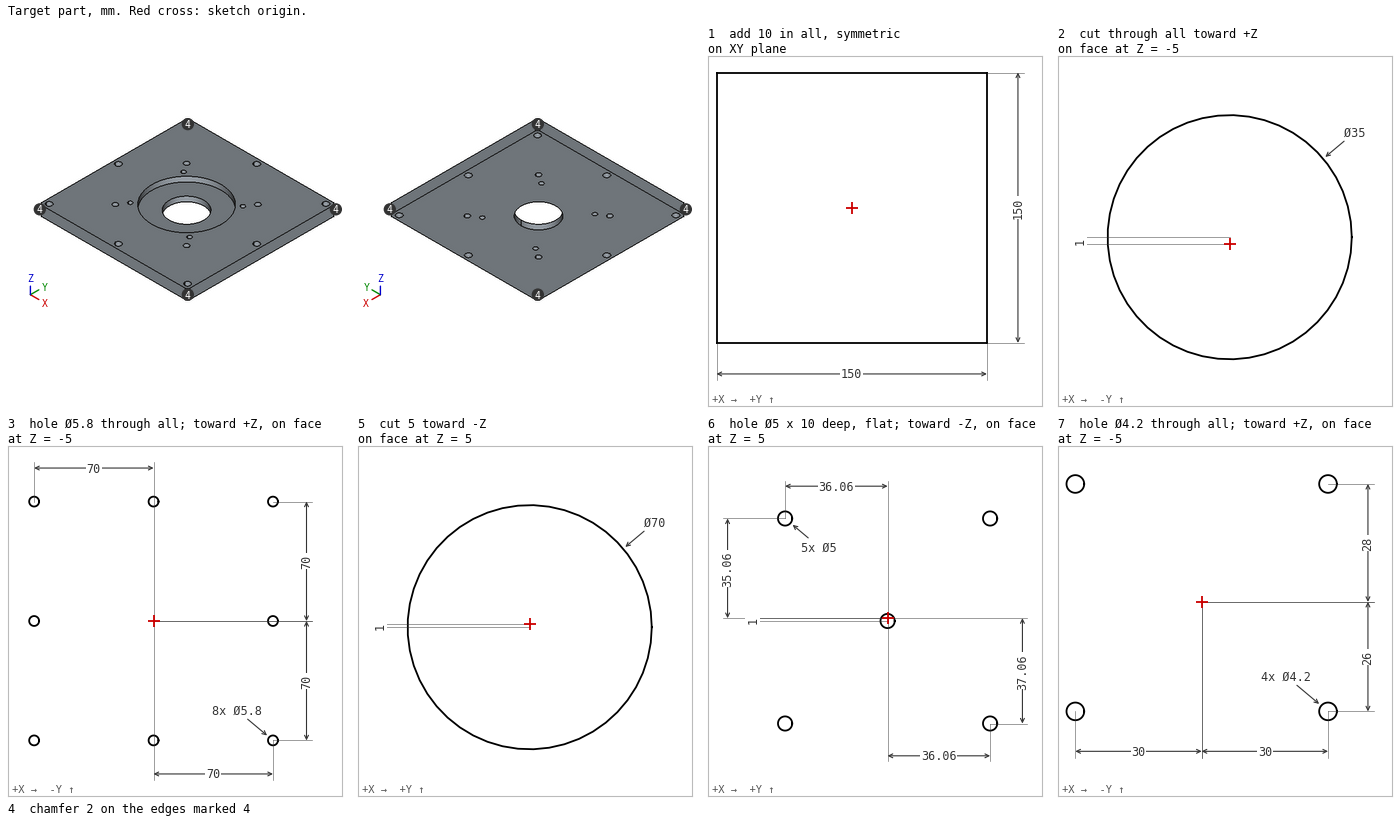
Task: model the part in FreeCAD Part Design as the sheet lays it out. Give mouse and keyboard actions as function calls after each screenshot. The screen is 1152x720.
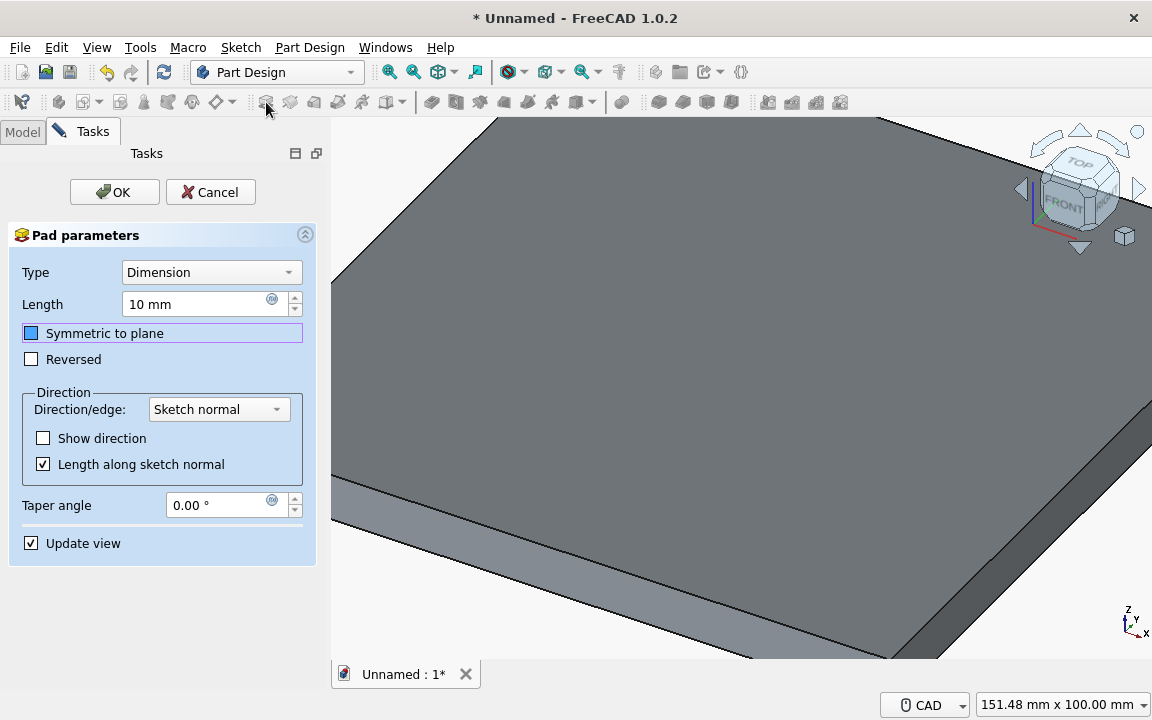
click(30, 333)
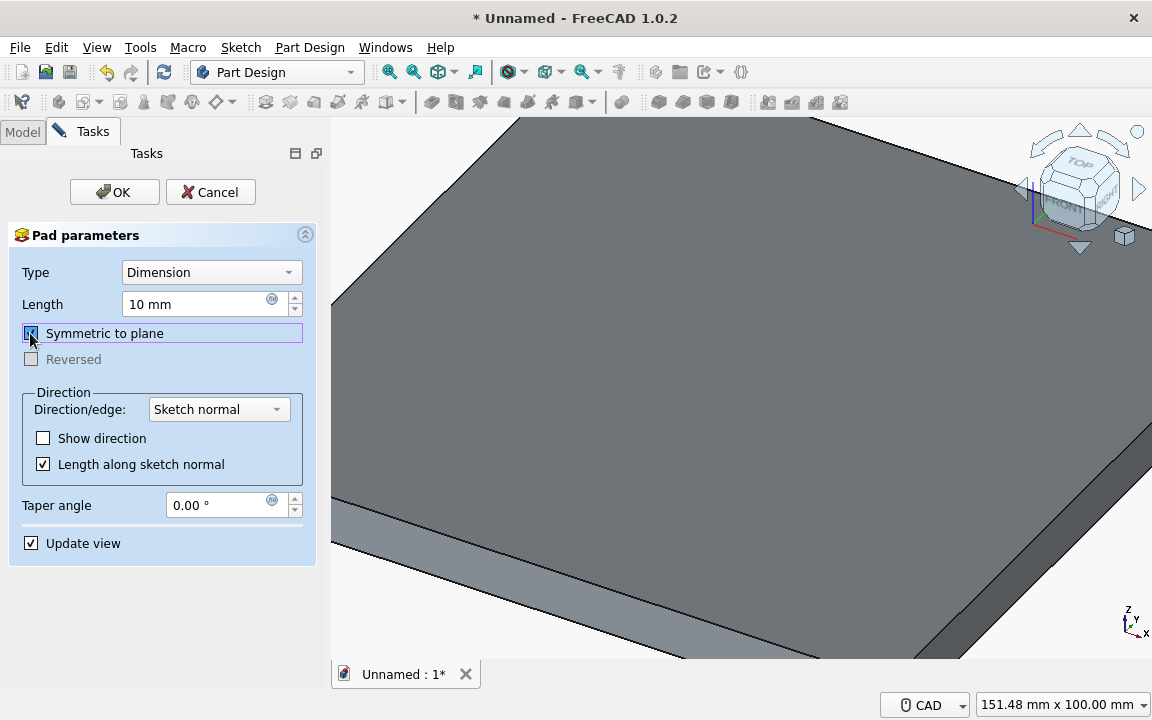
click(115, 192)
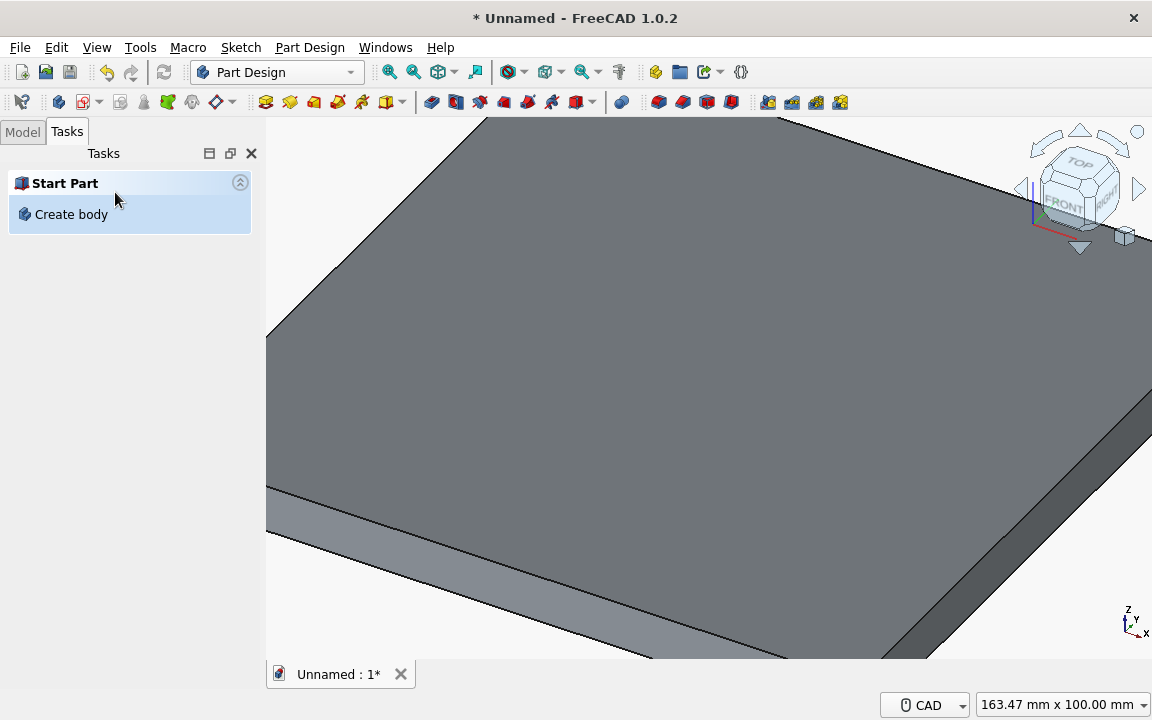
key(v)
key(f)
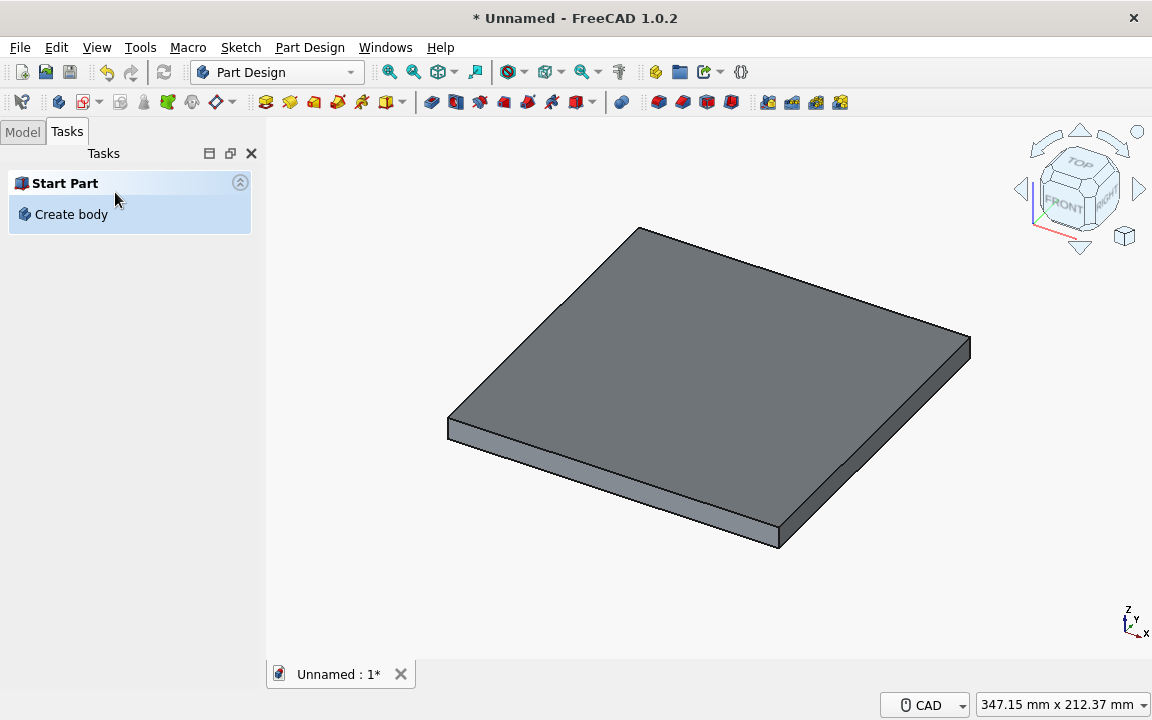
key(5)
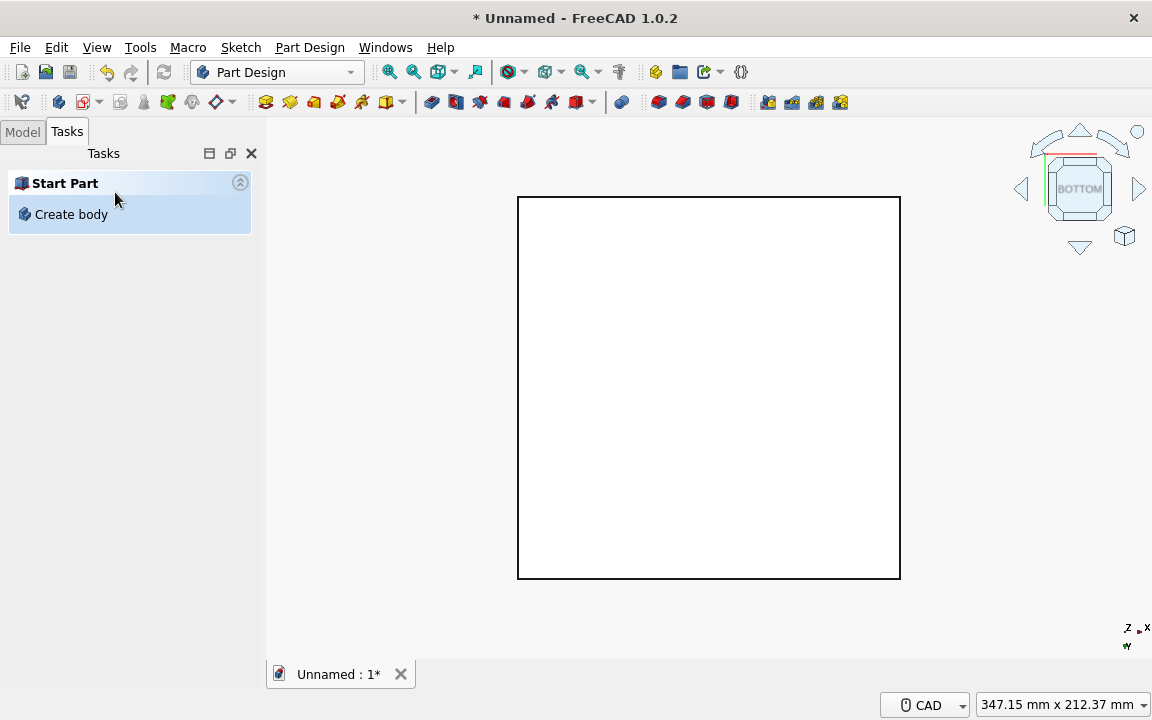
click(709, 387)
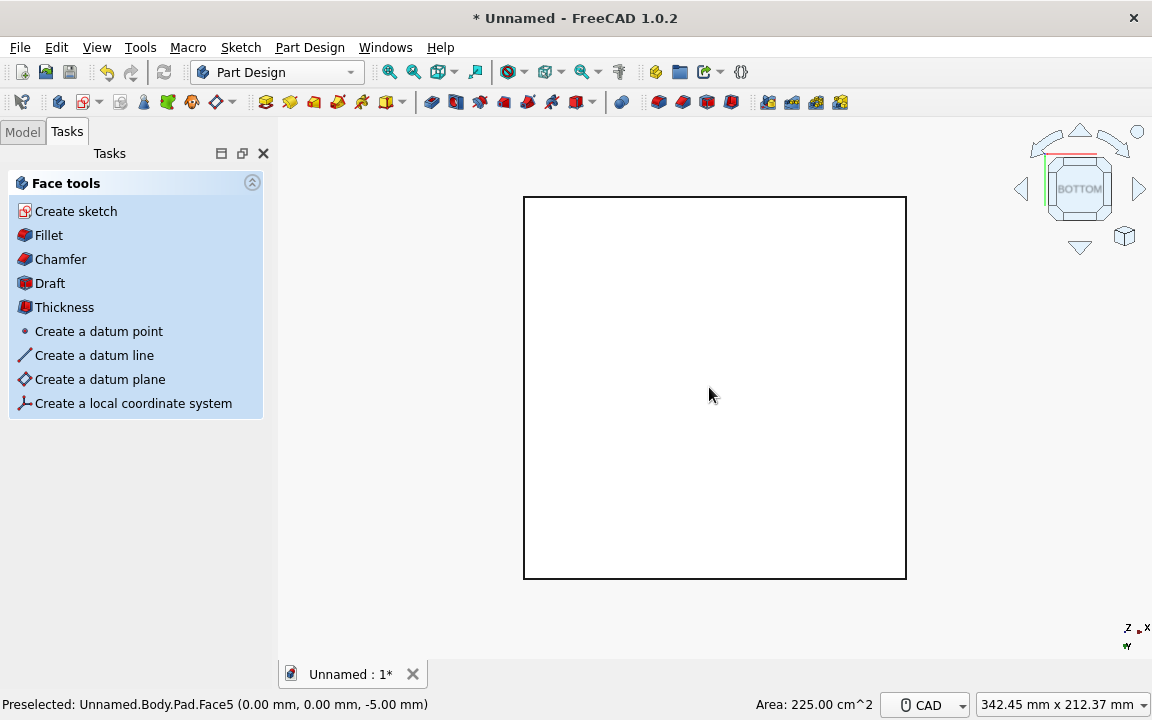
click(84, 102)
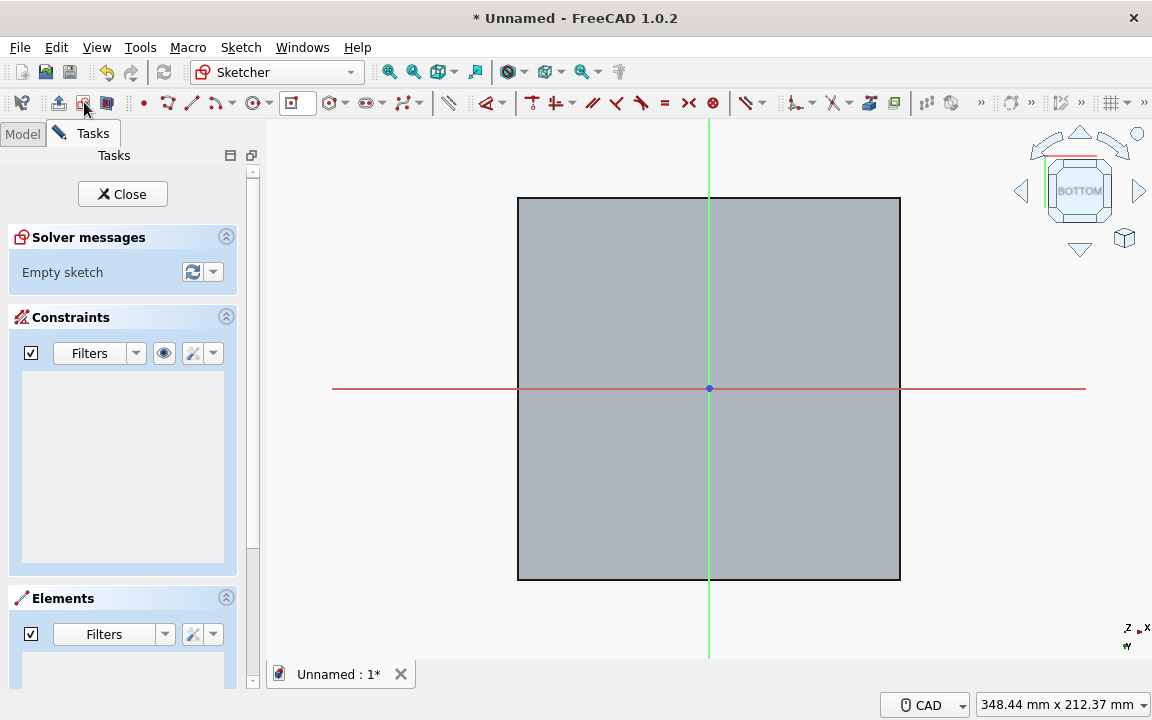
scroll(731, 386, up, 7)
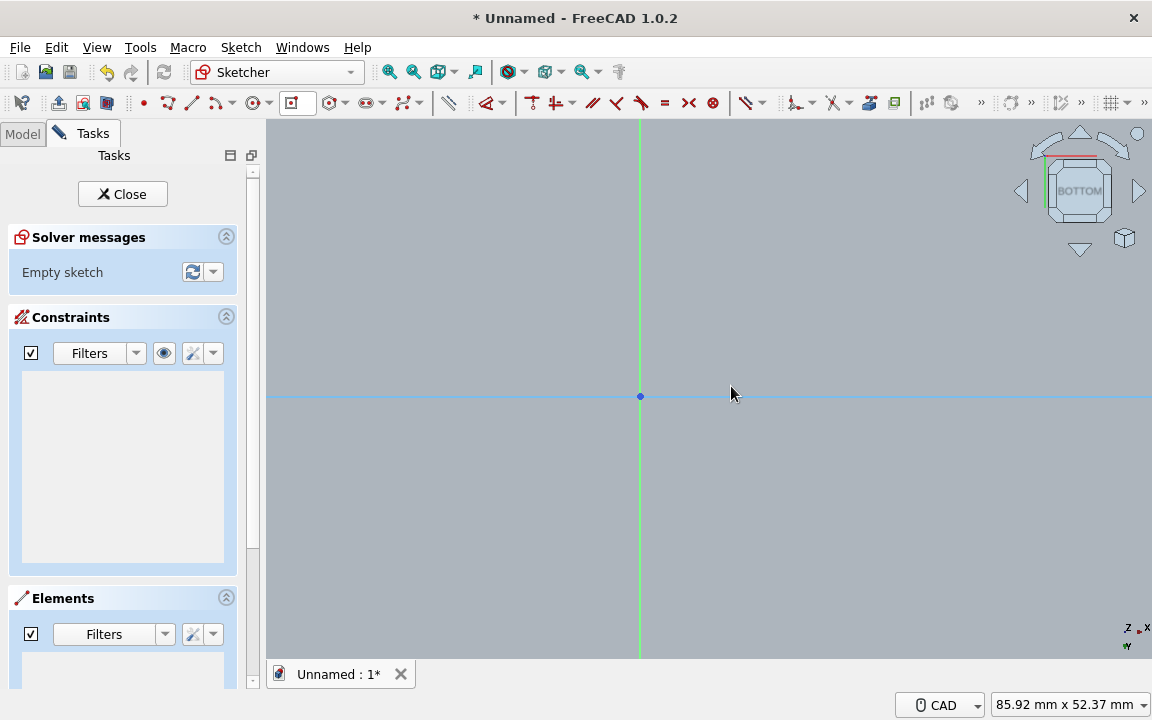
click(254, 104)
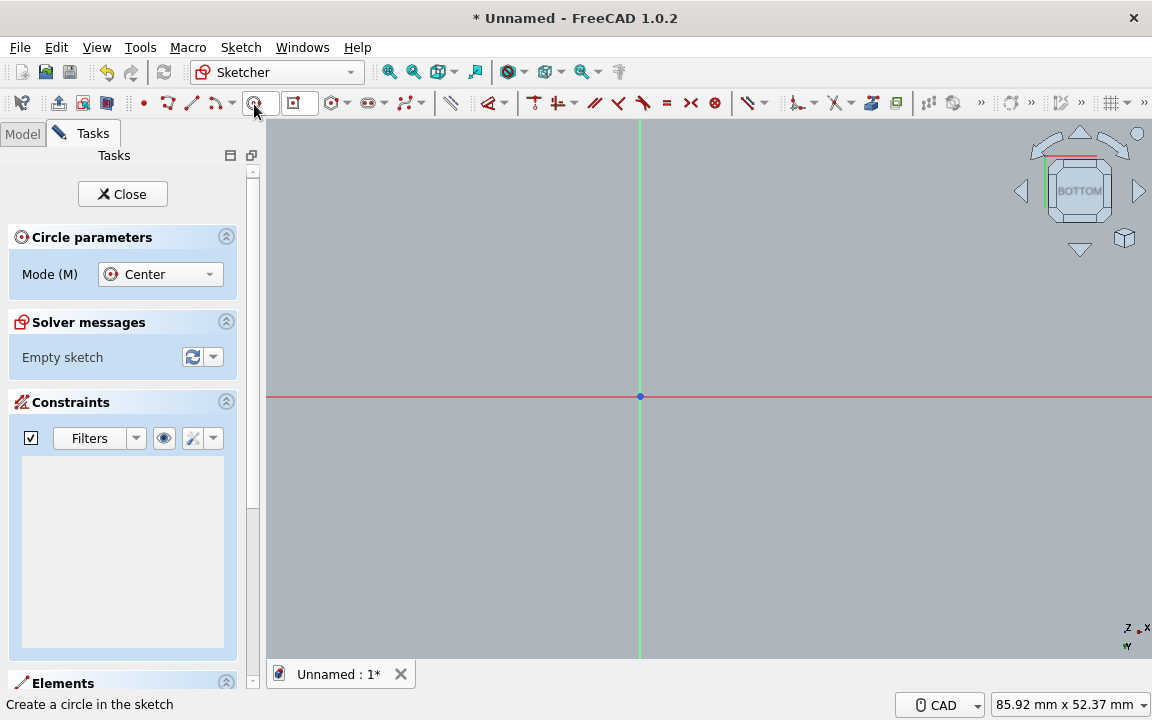
scroll(640, 386, up, 3)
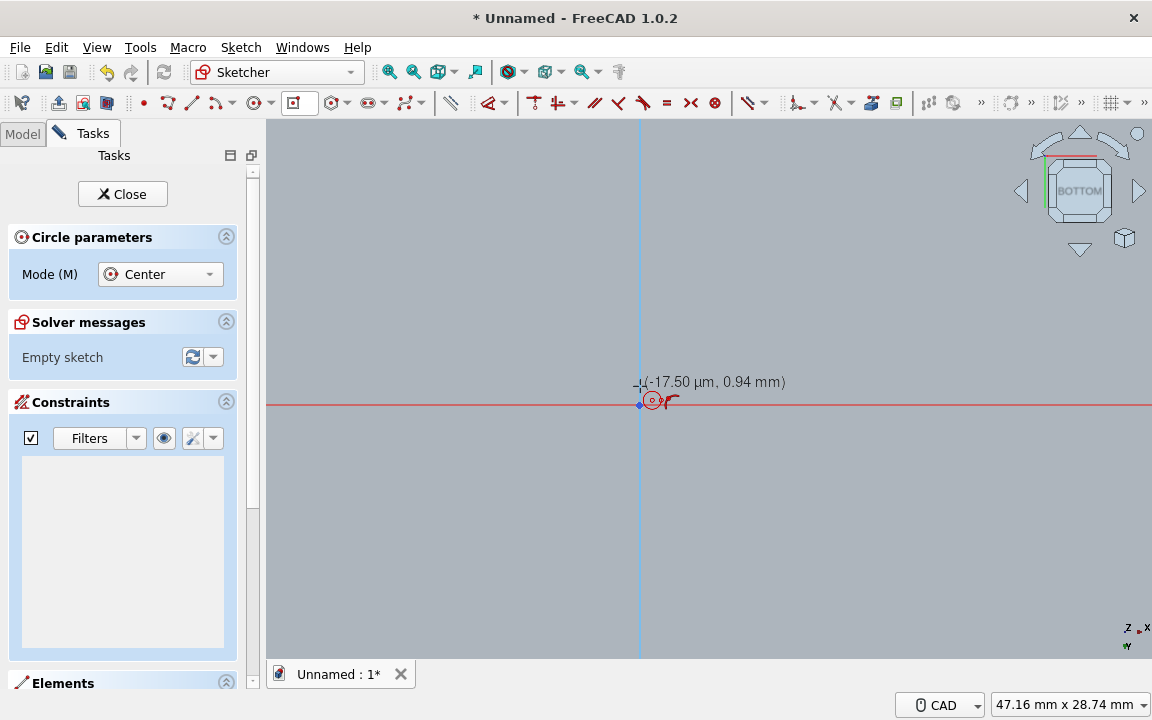
click(640, 386)
move(872, 154)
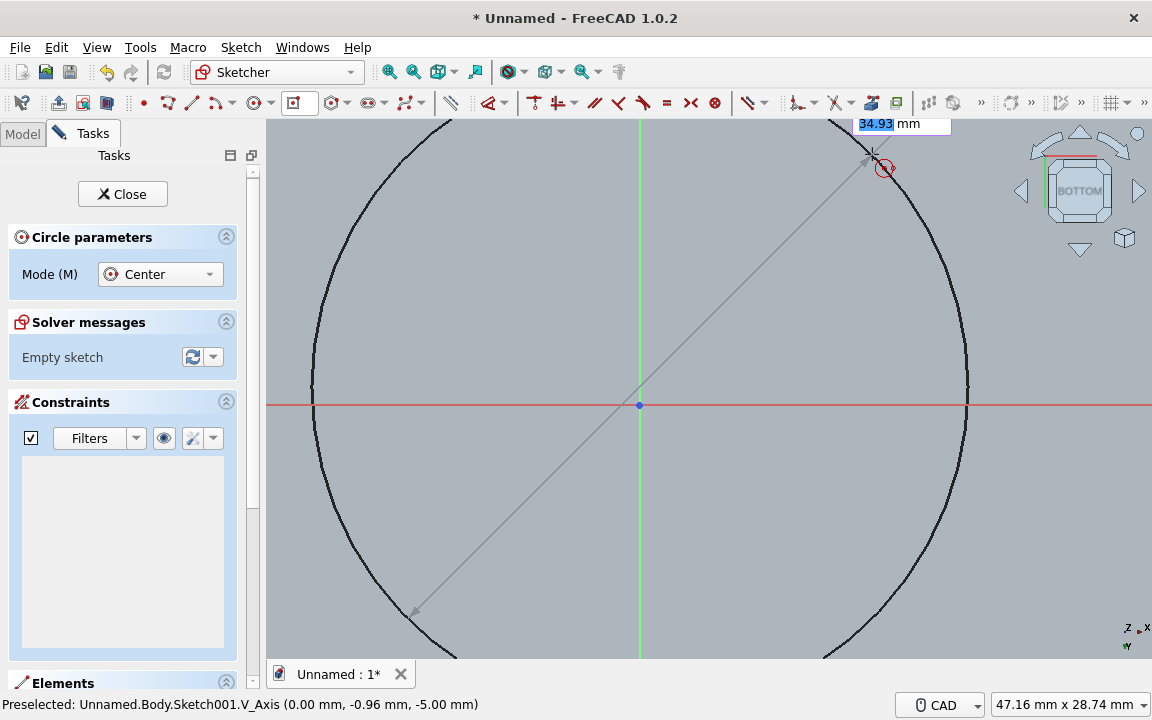
text(35)
key(Return)
key(Escape)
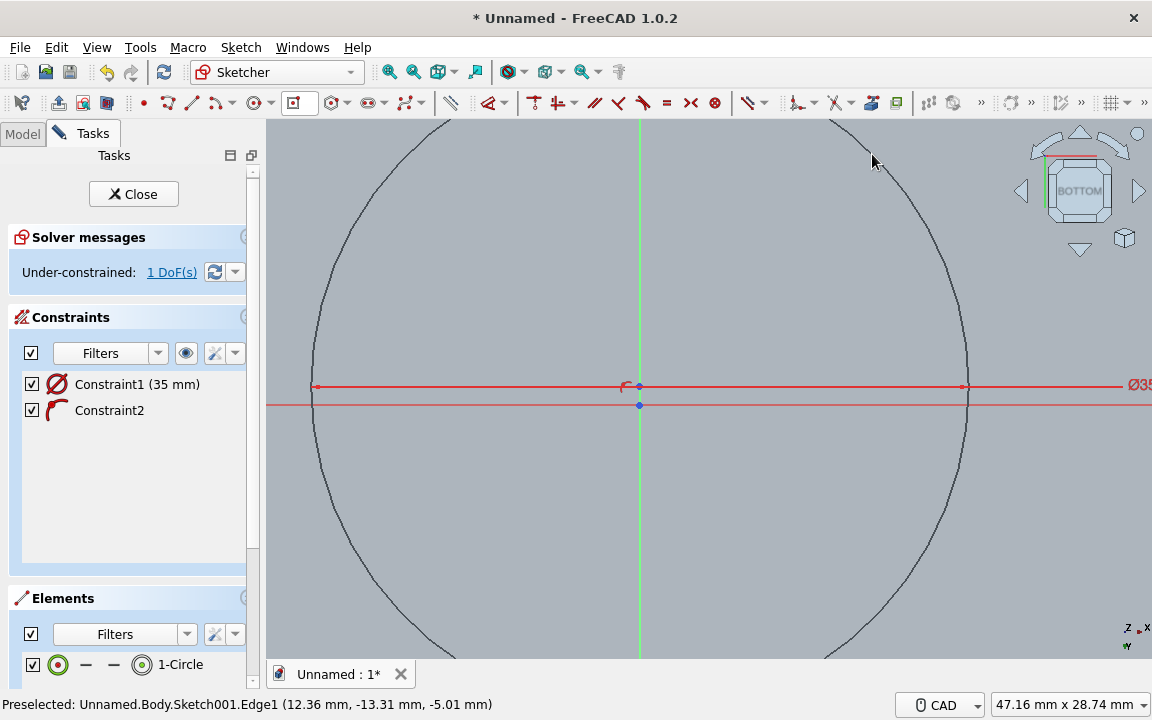
click(488, 104)